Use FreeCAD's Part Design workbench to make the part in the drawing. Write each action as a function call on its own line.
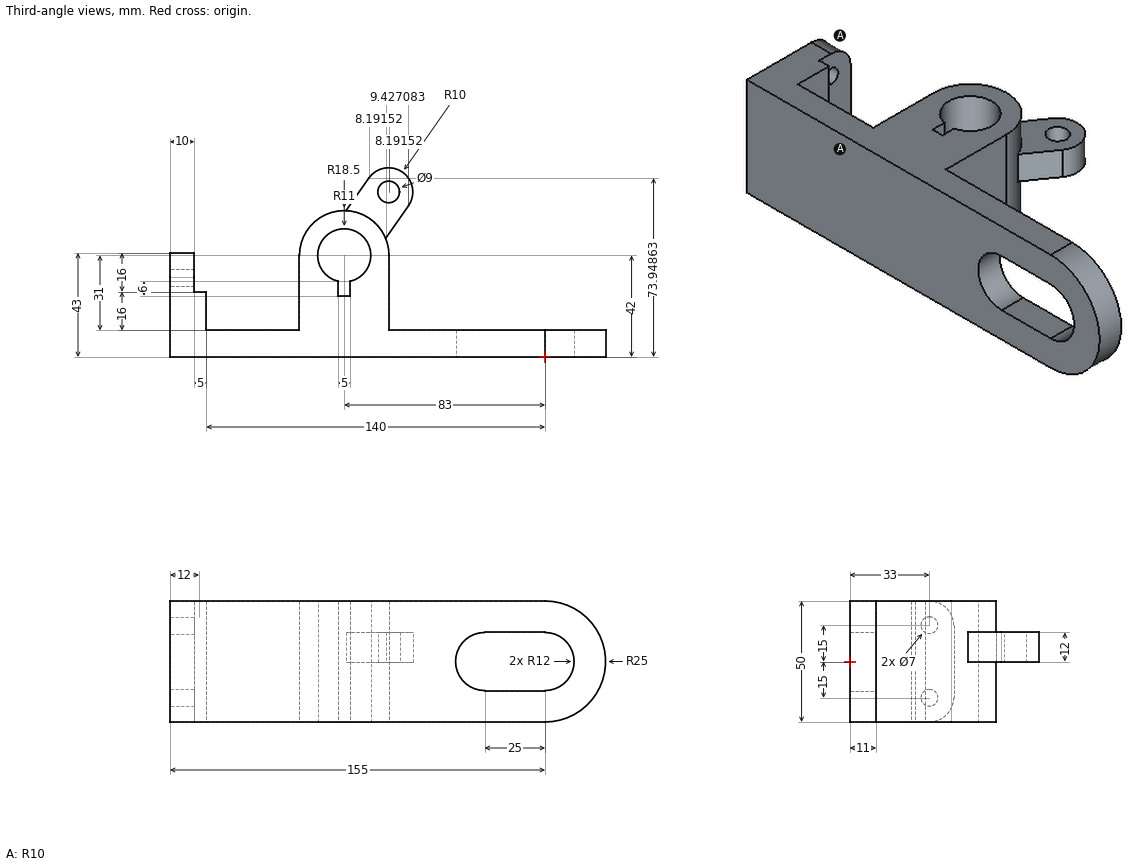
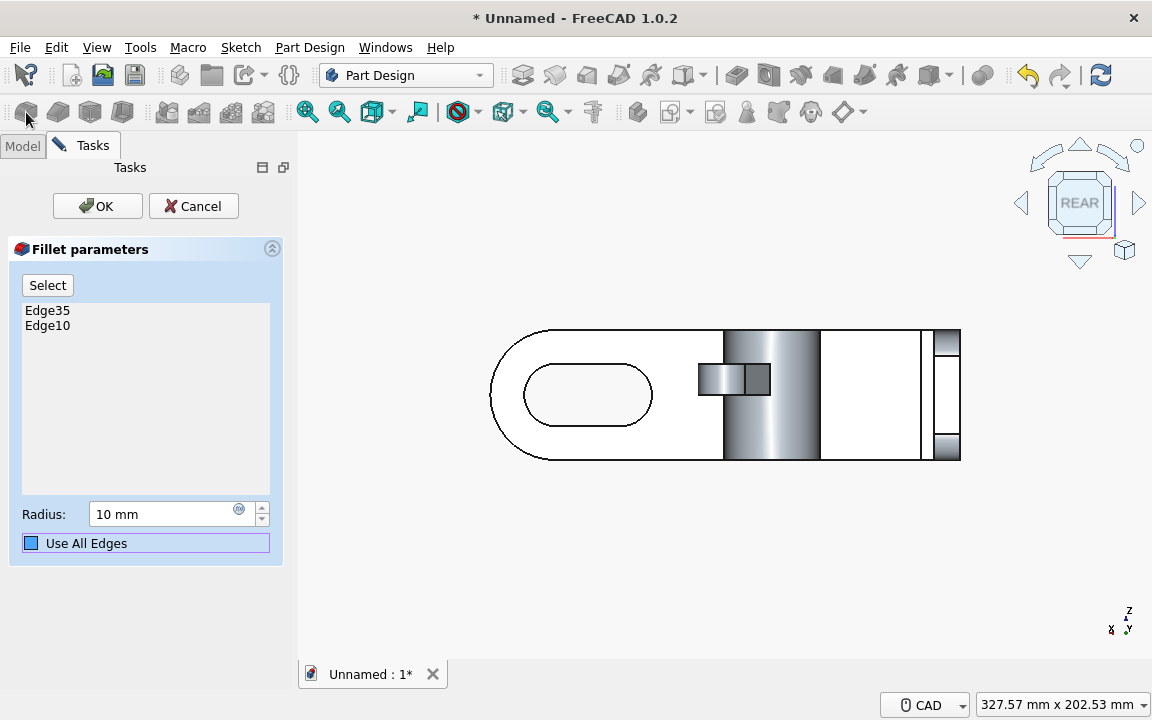
click(98, 206)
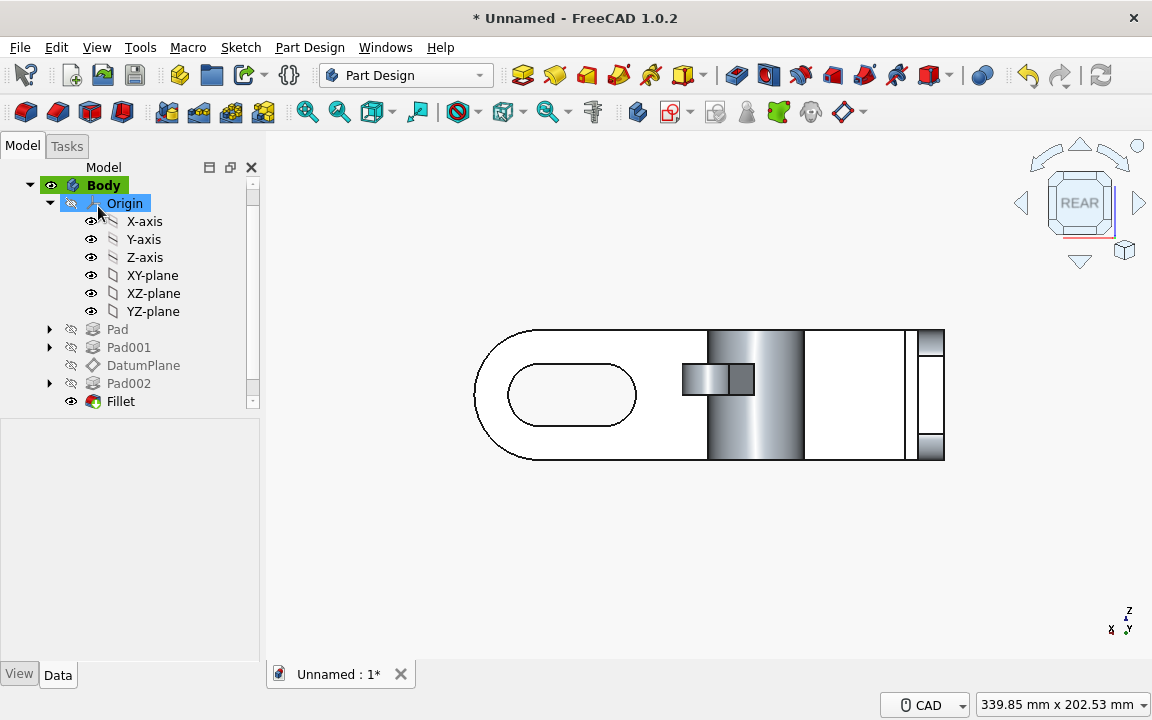
key(6)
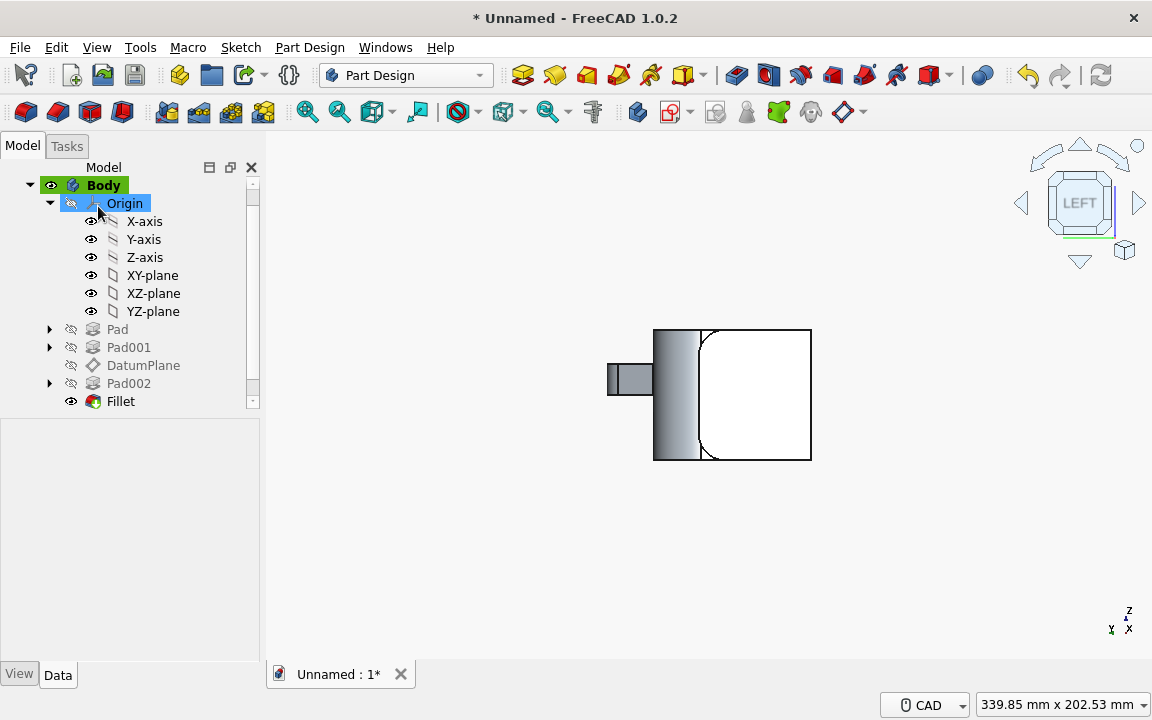
key(v)
key(f)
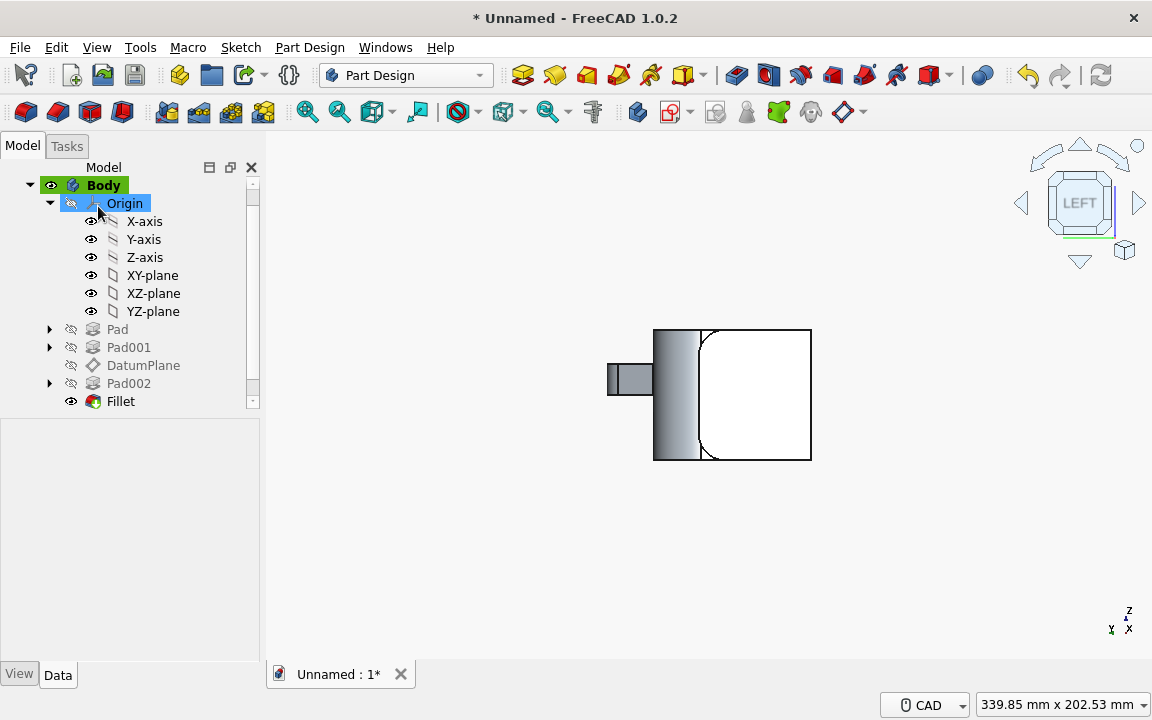
click(755, 394)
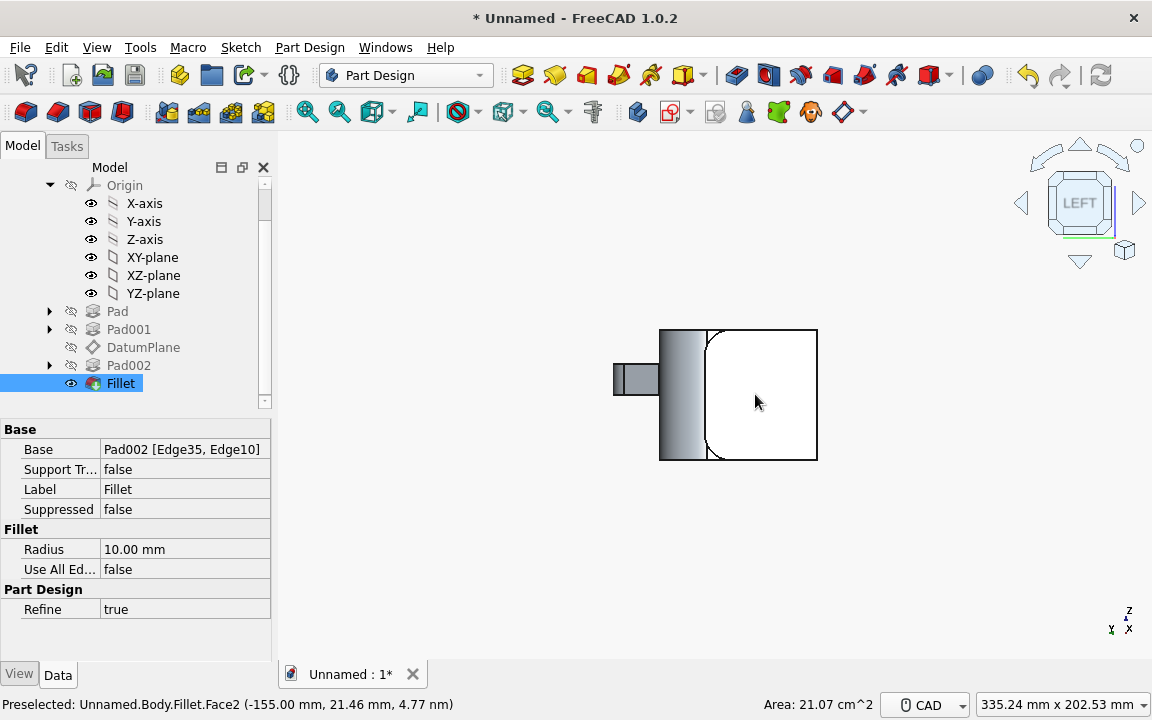
click(670, 112)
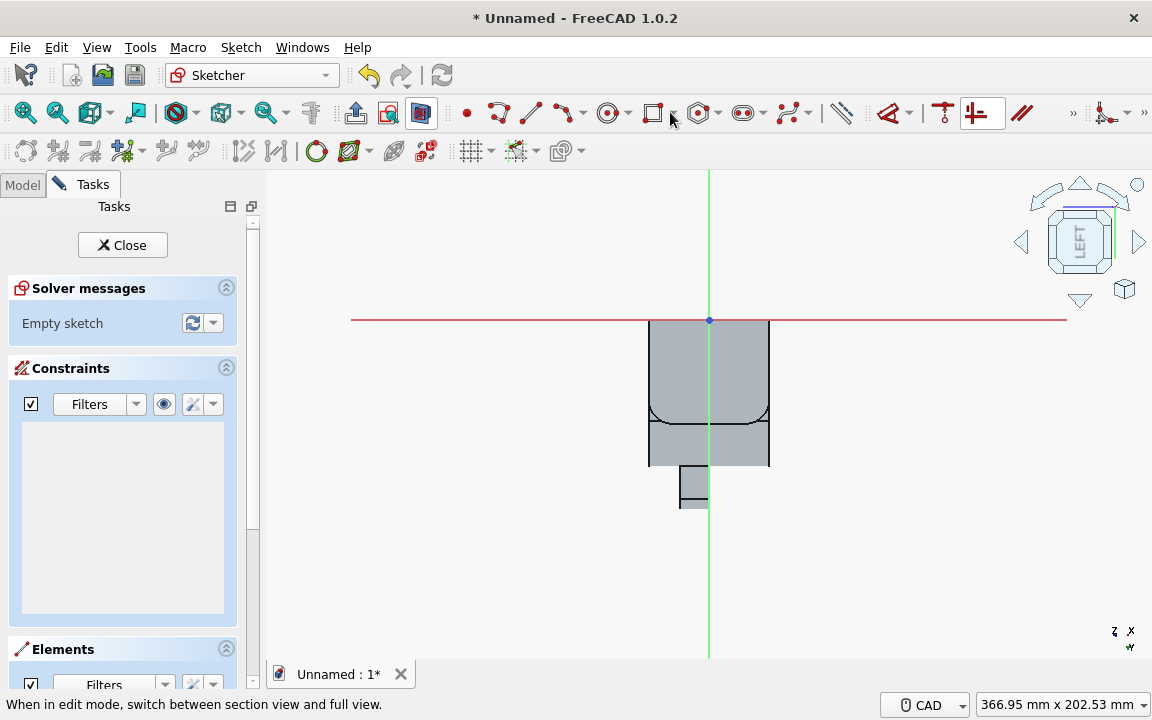
scroll(739, 342, up, 6)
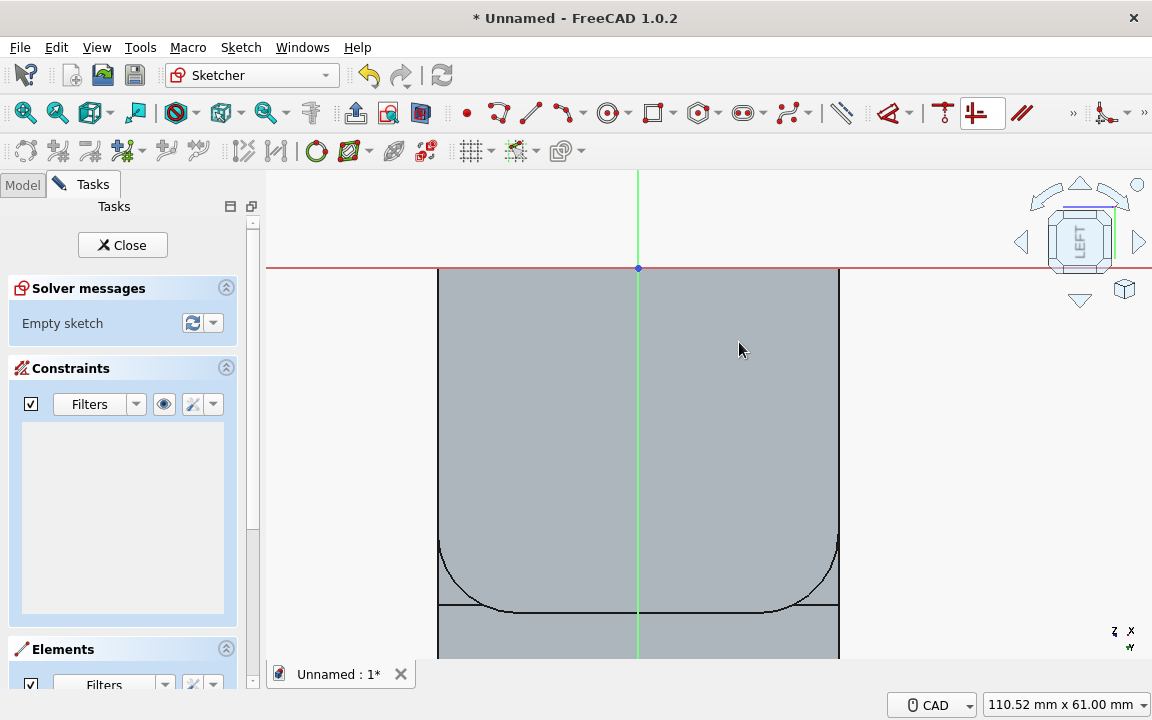
click(608, 114)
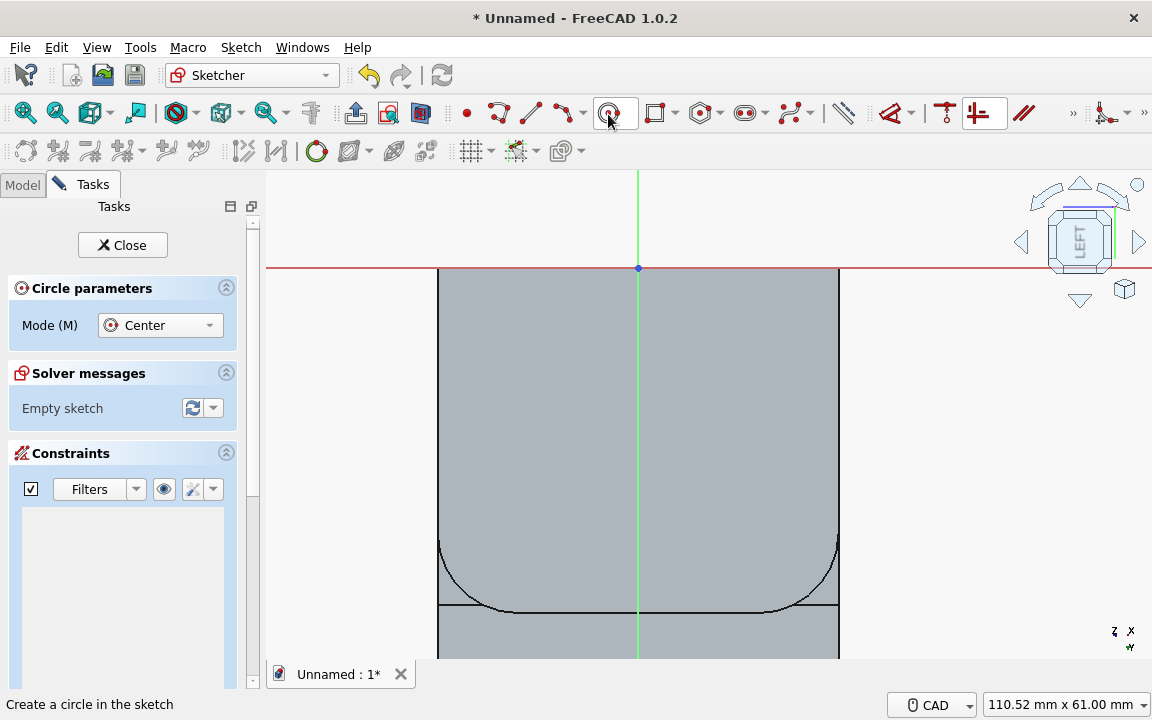
click(518, 533)
move(538, 513)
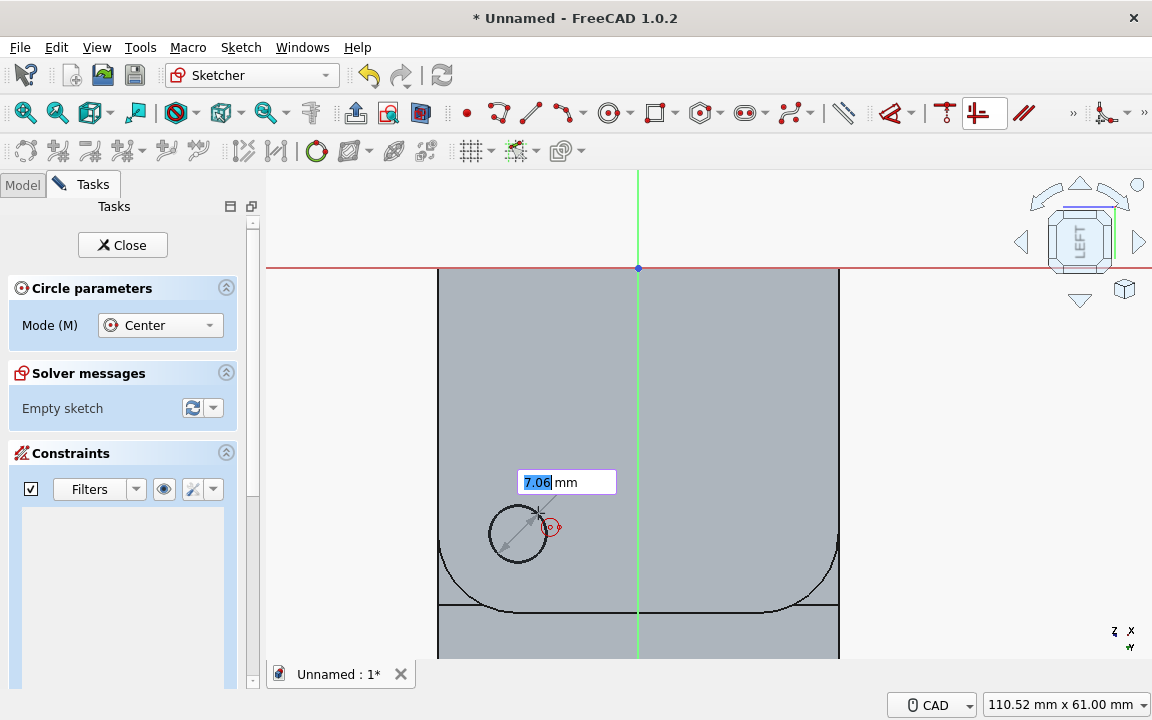
text(7)
key(Return)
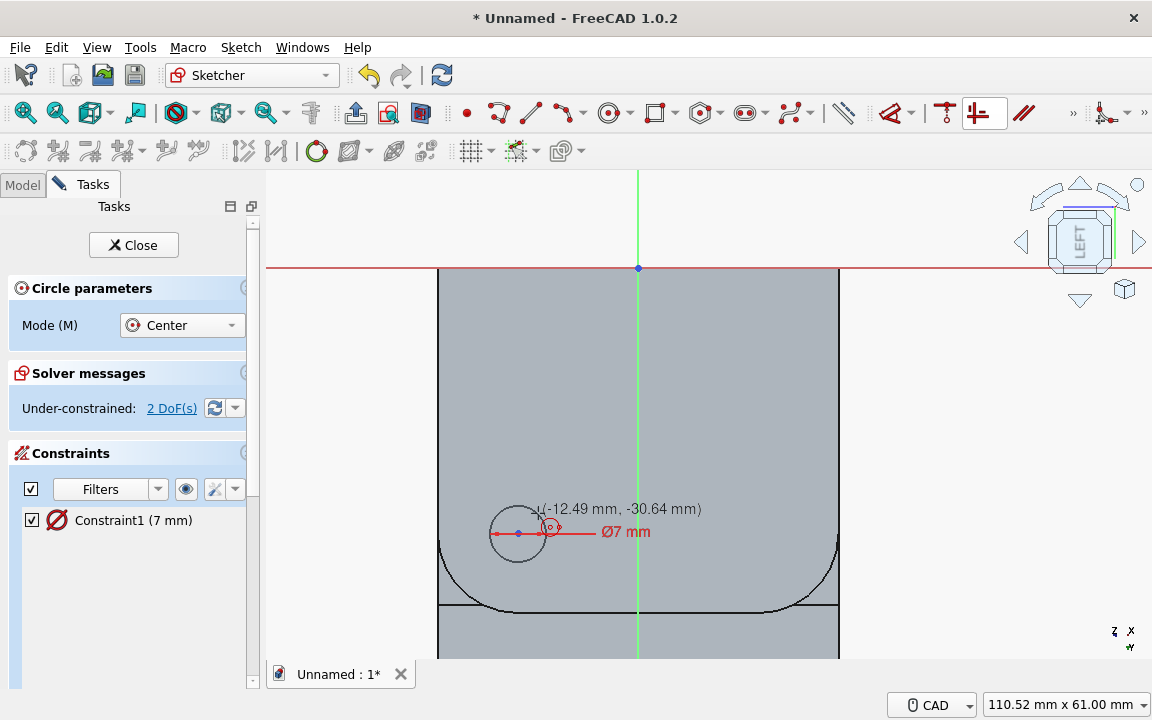
click(758, 533)
move(778, 513)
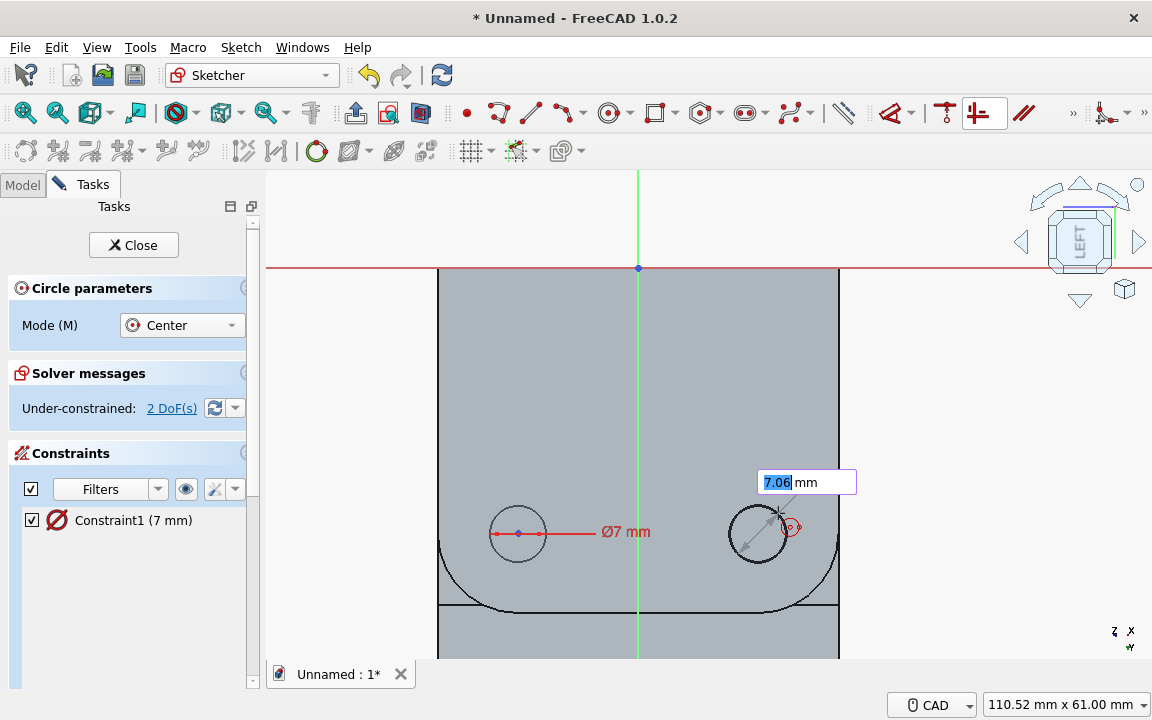
text(7)
key(Return)
key(Escape)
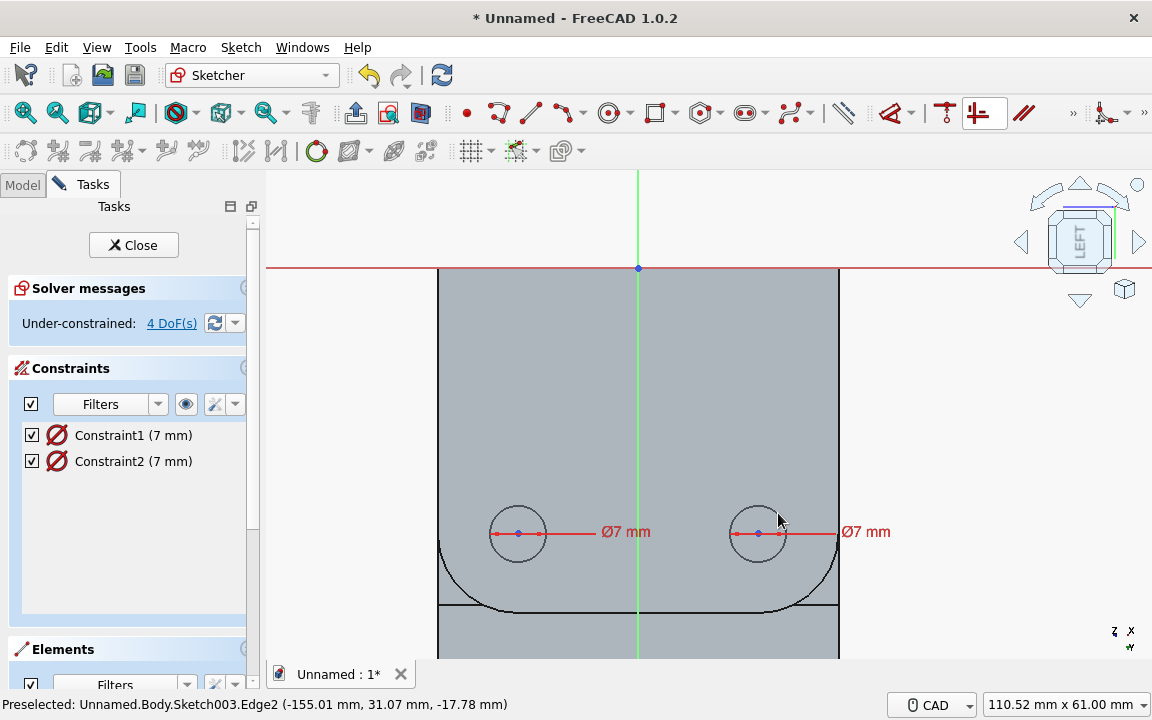
click(518, 534)